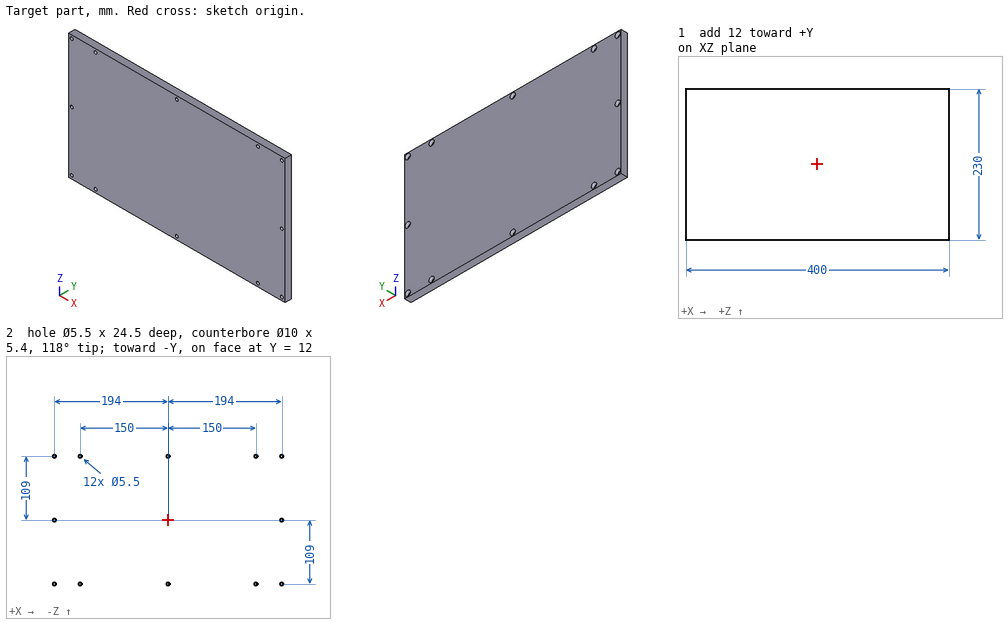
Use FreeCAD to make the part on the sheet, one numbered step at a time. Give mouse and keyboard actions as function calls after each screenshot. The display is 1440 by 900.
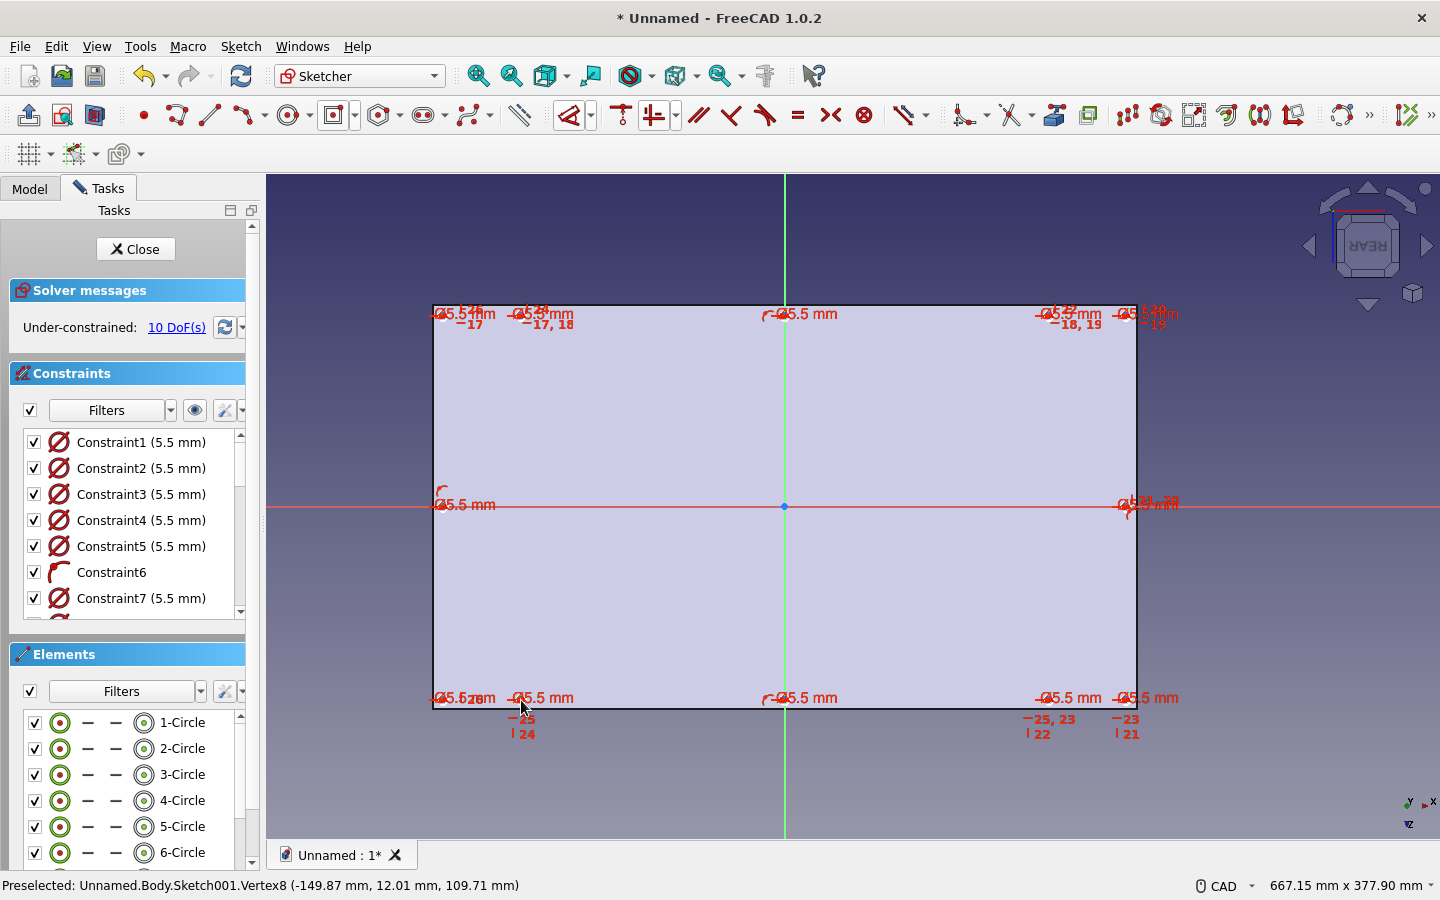
click(443, 700)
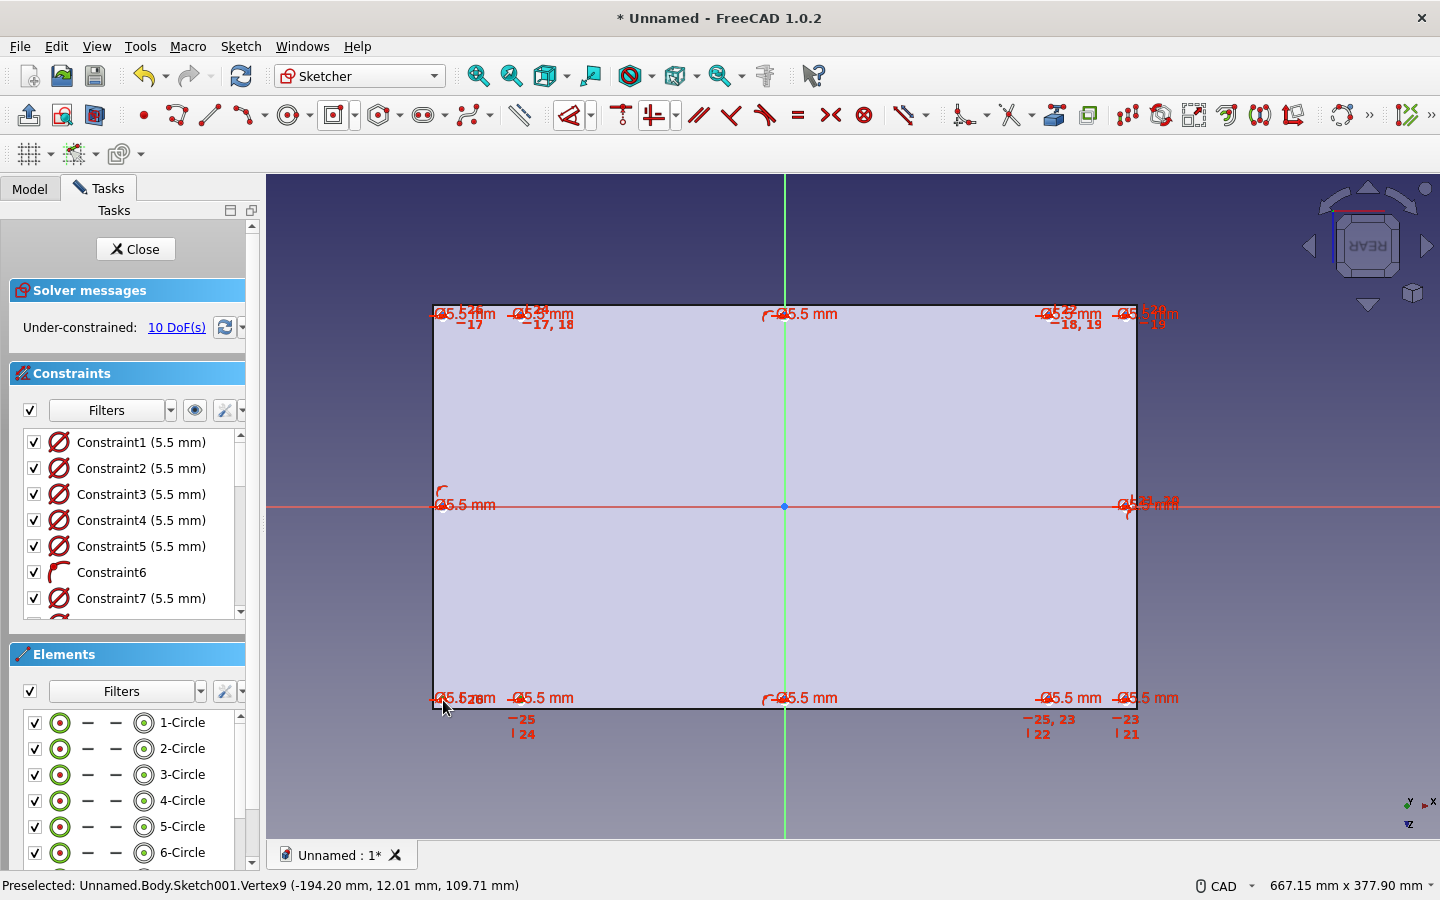
key(h)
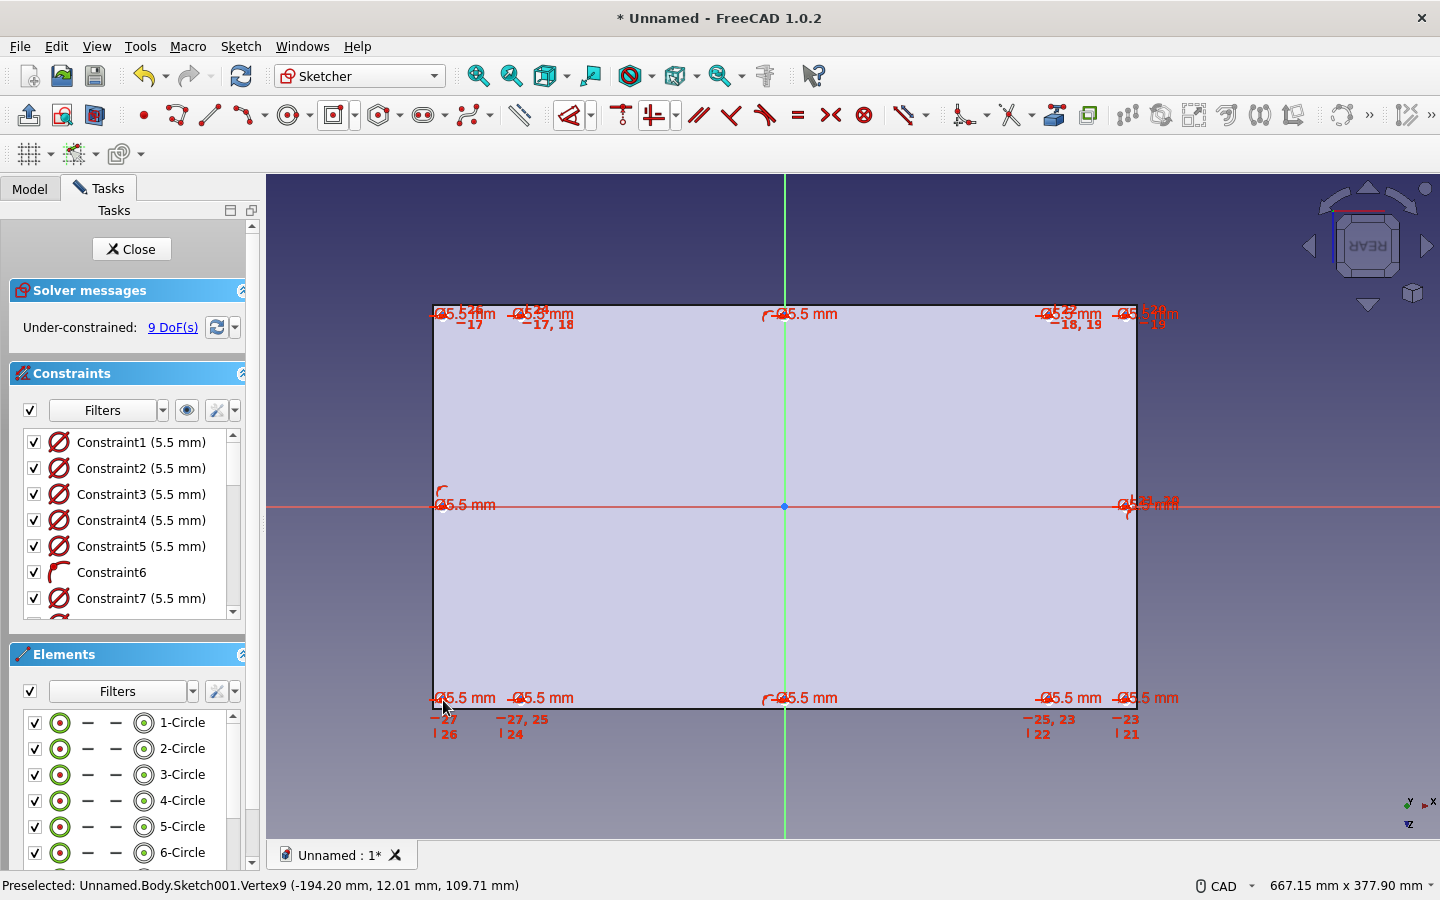
click(443, 316)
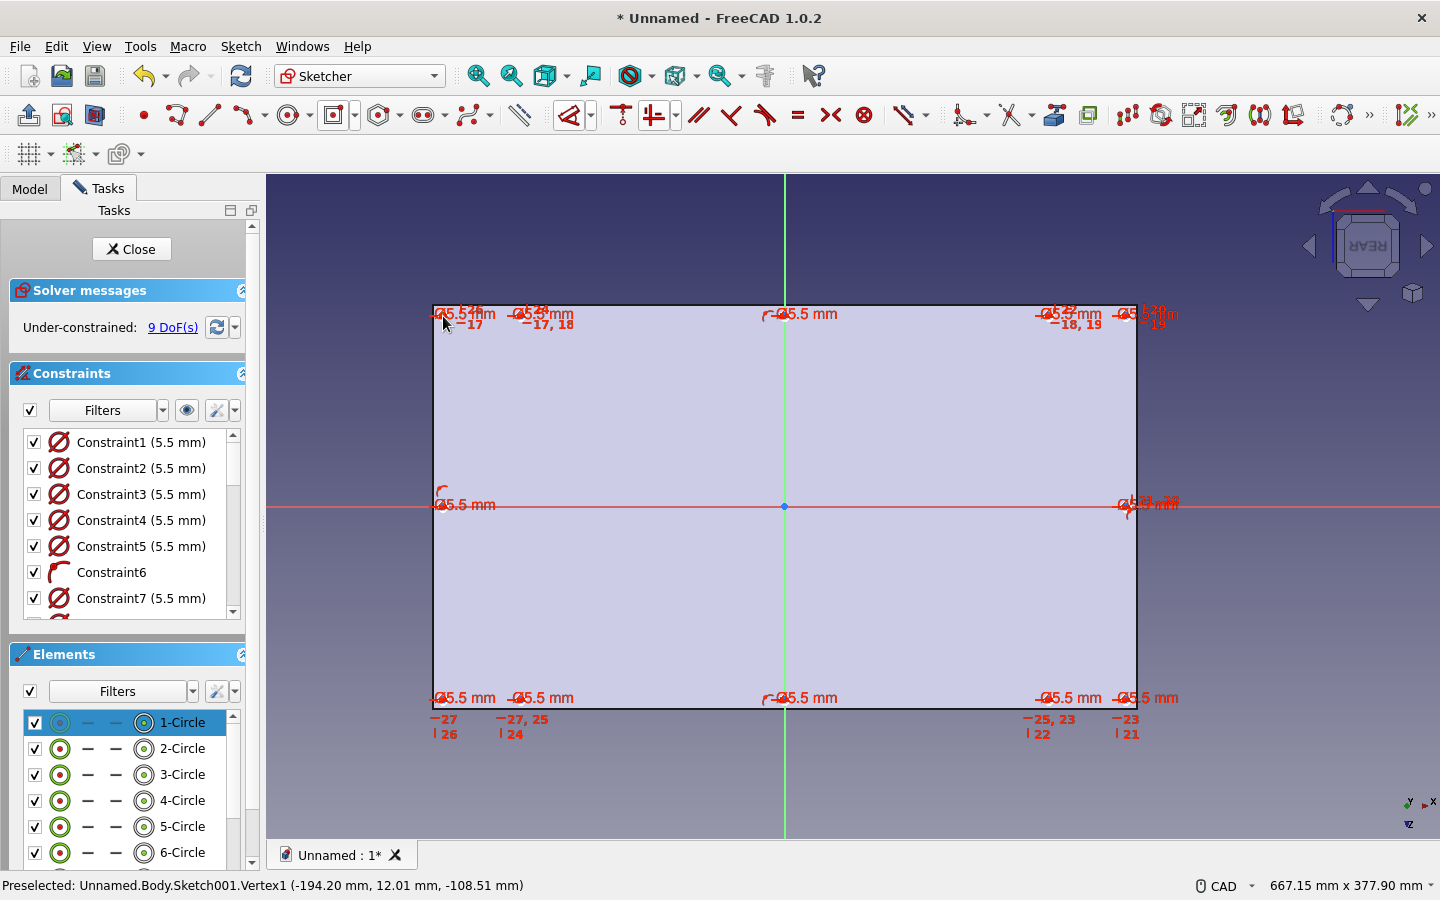
click(443, 507)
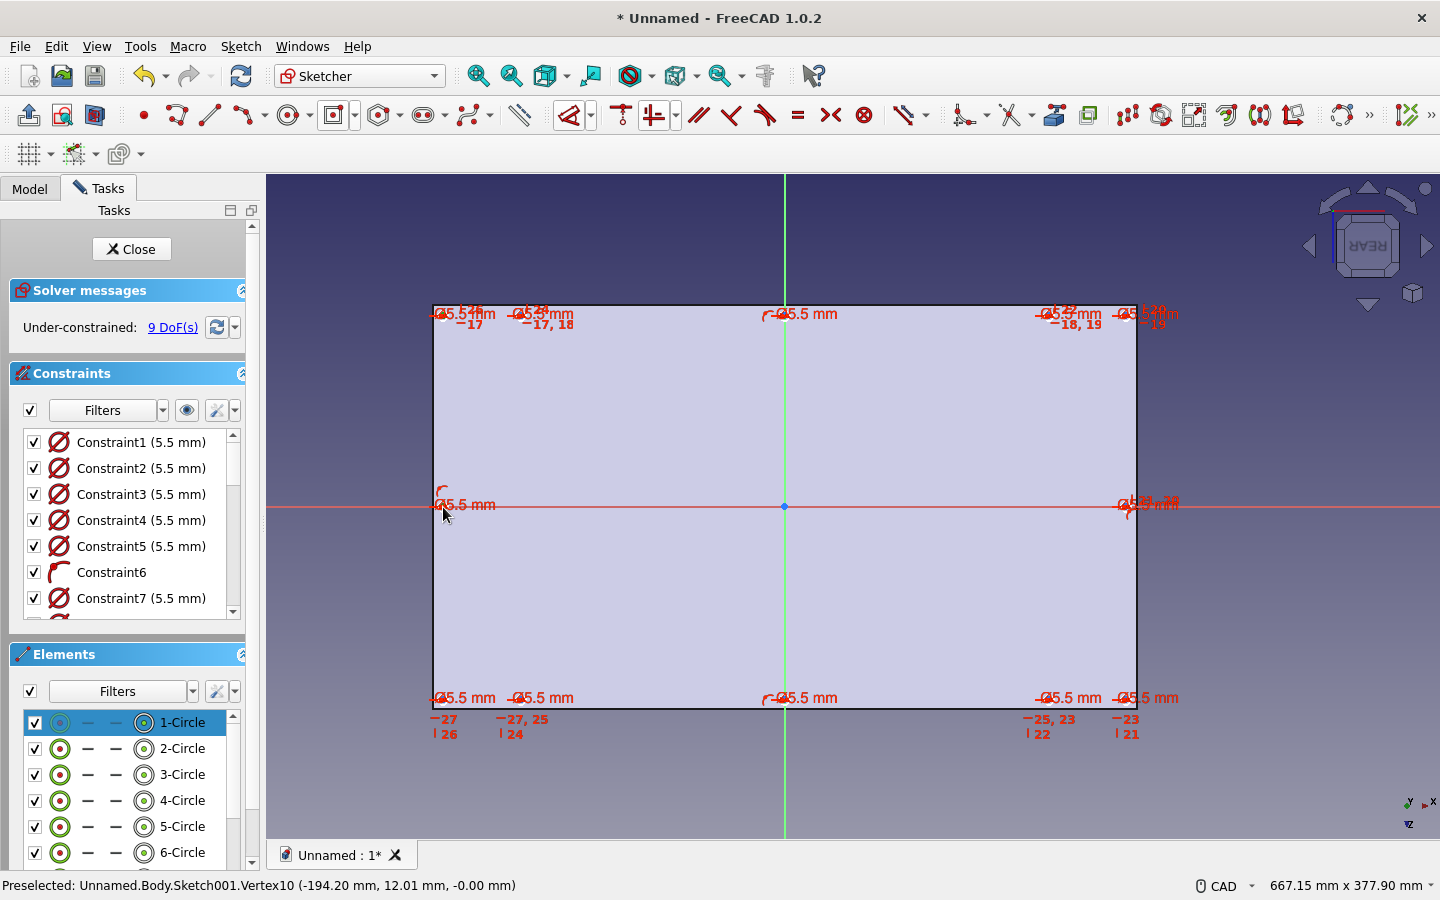
click(676, 116)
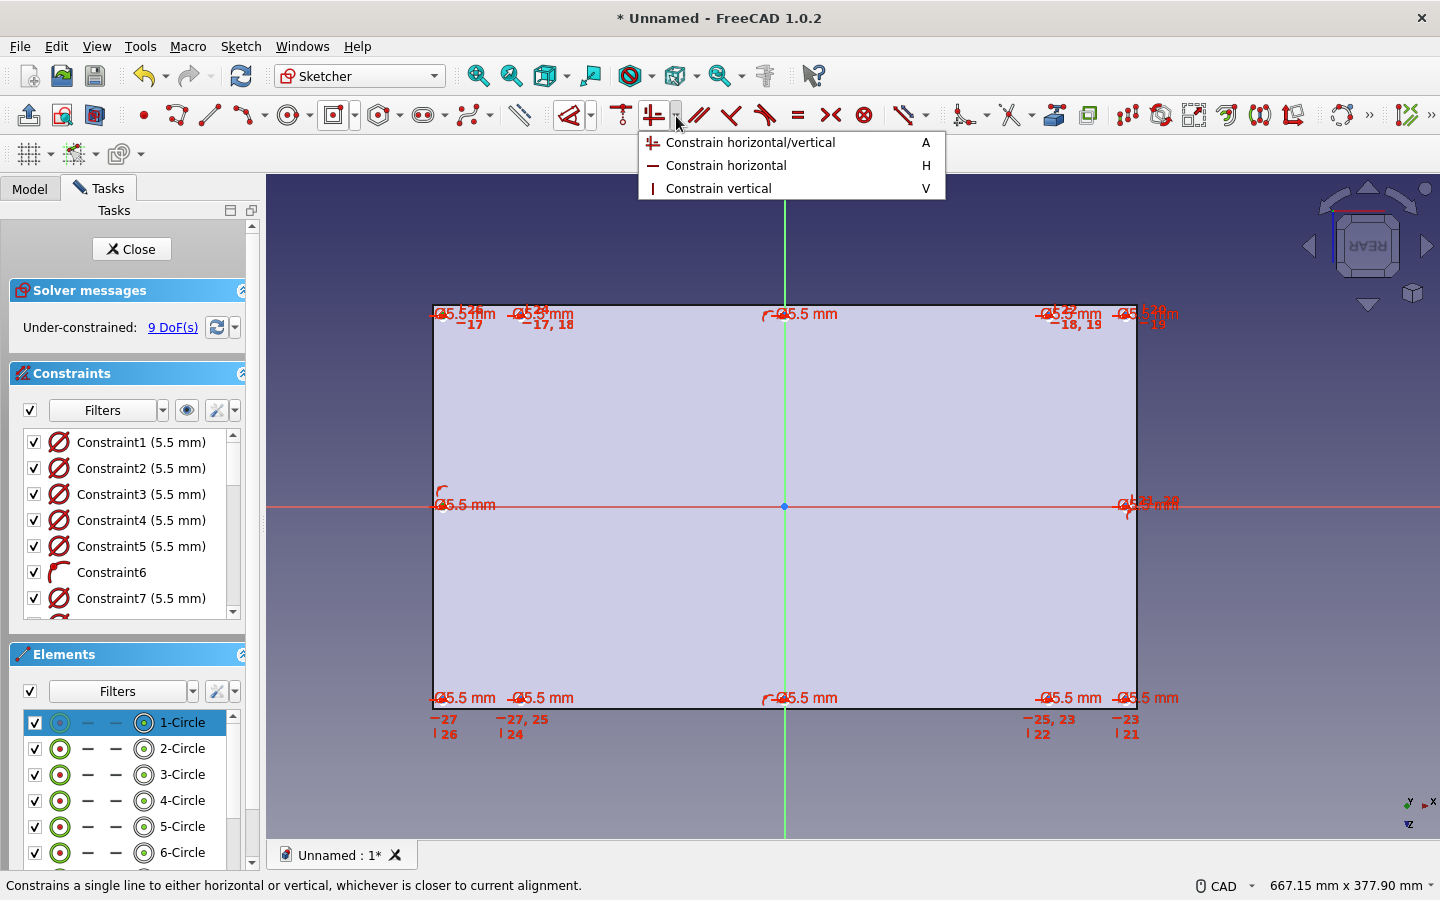
click(792, 188)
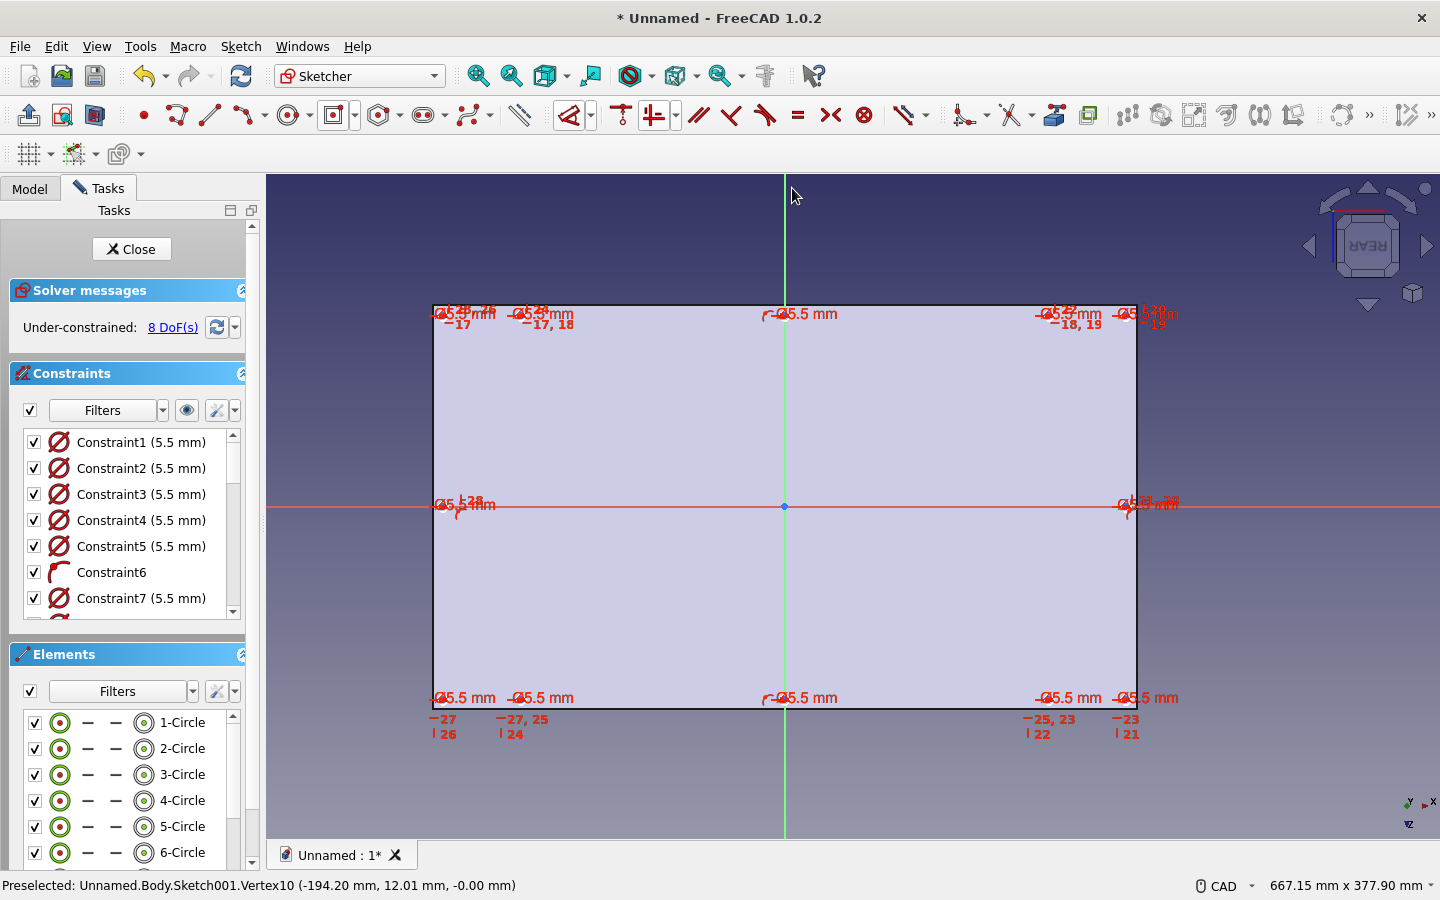
click(521, 316)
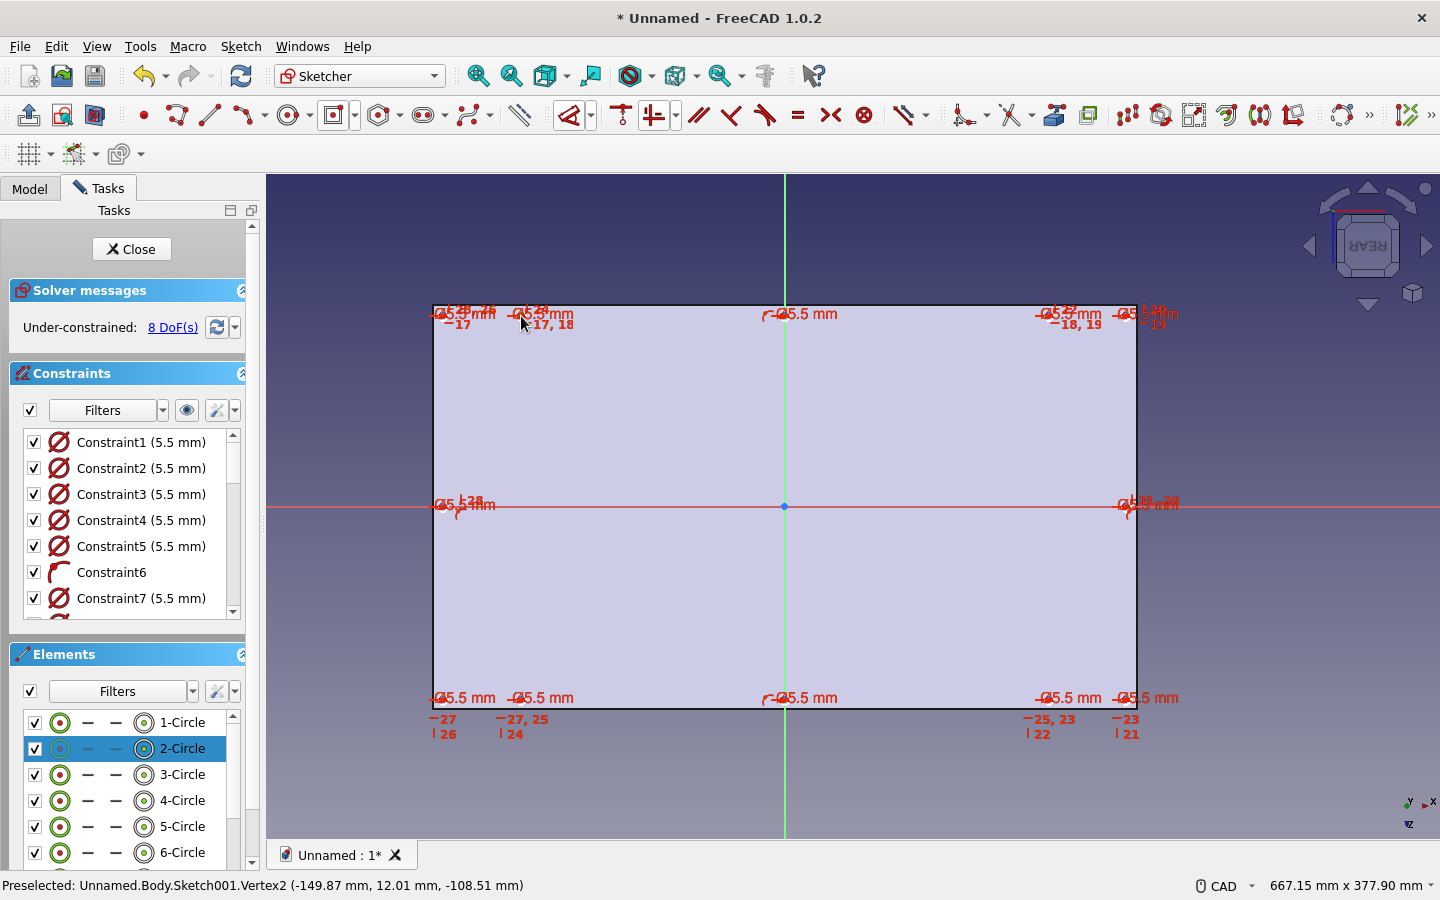
click(785, 316)